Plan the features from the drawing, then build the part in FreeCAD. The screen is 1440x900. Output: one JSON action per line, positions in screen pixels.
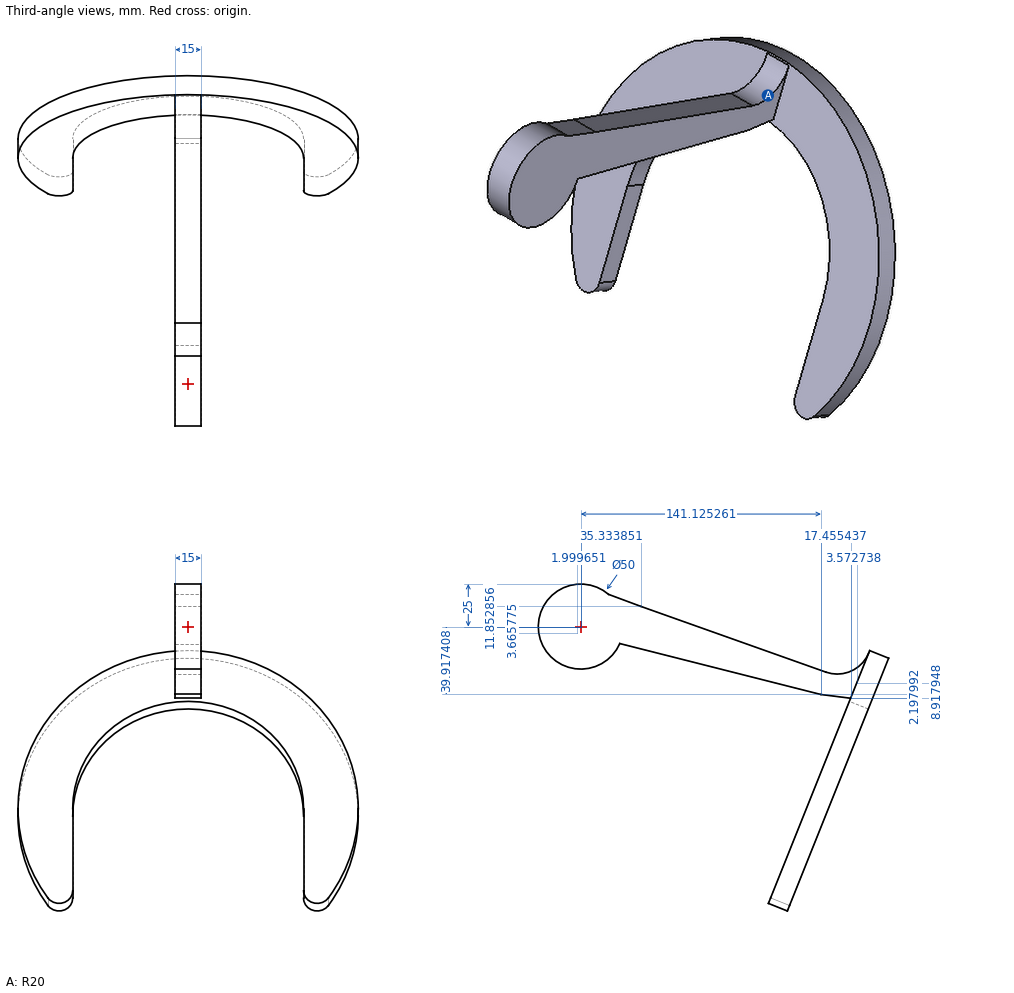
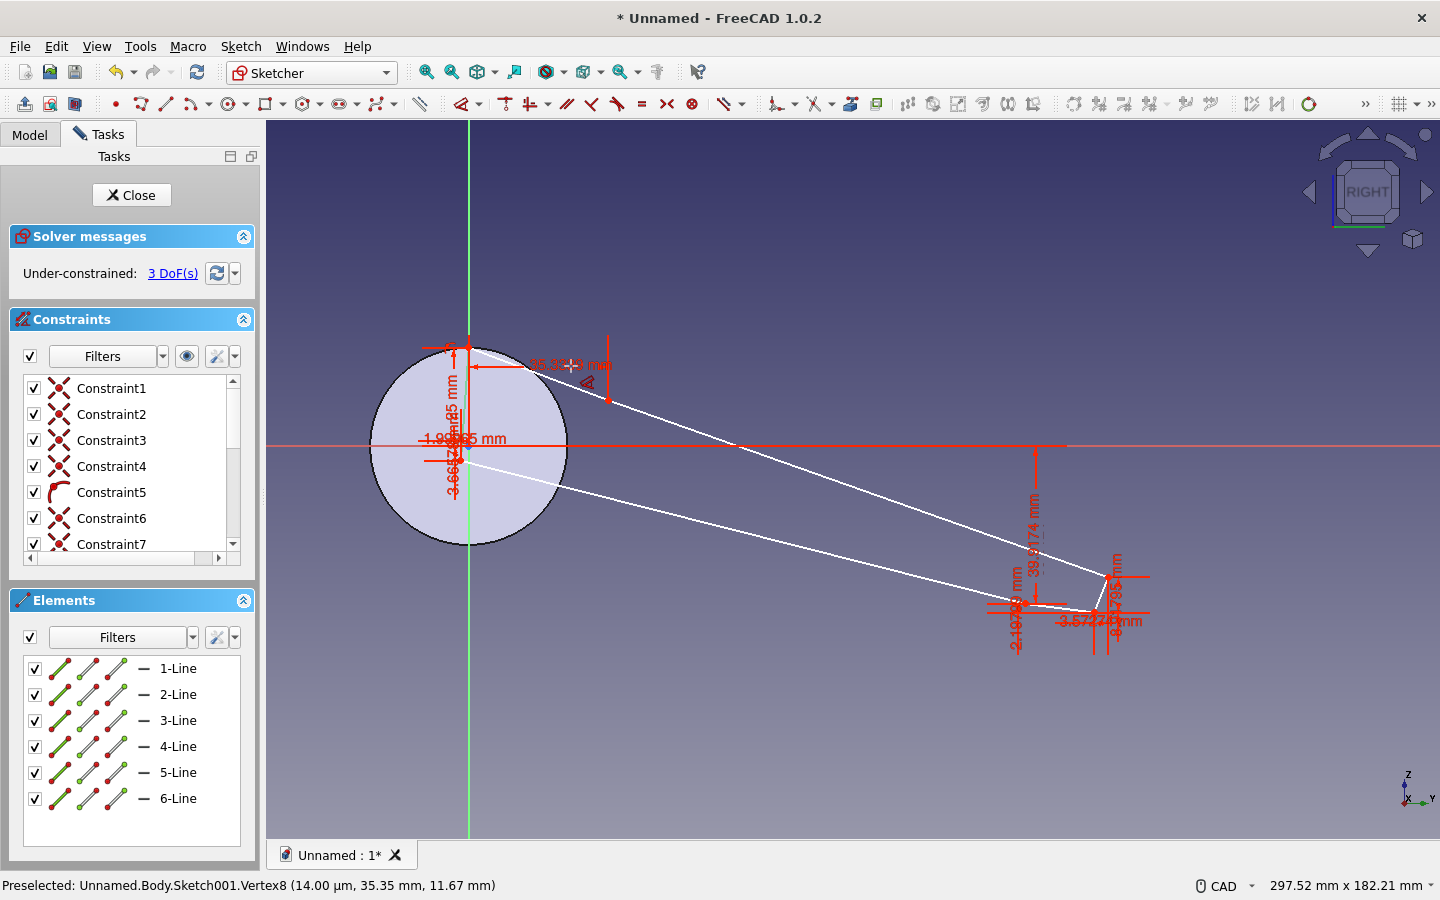
{"action": "left_click", "coordinate": [608, 400]}
{"action": "left_click", "coordinate": [387, 423]}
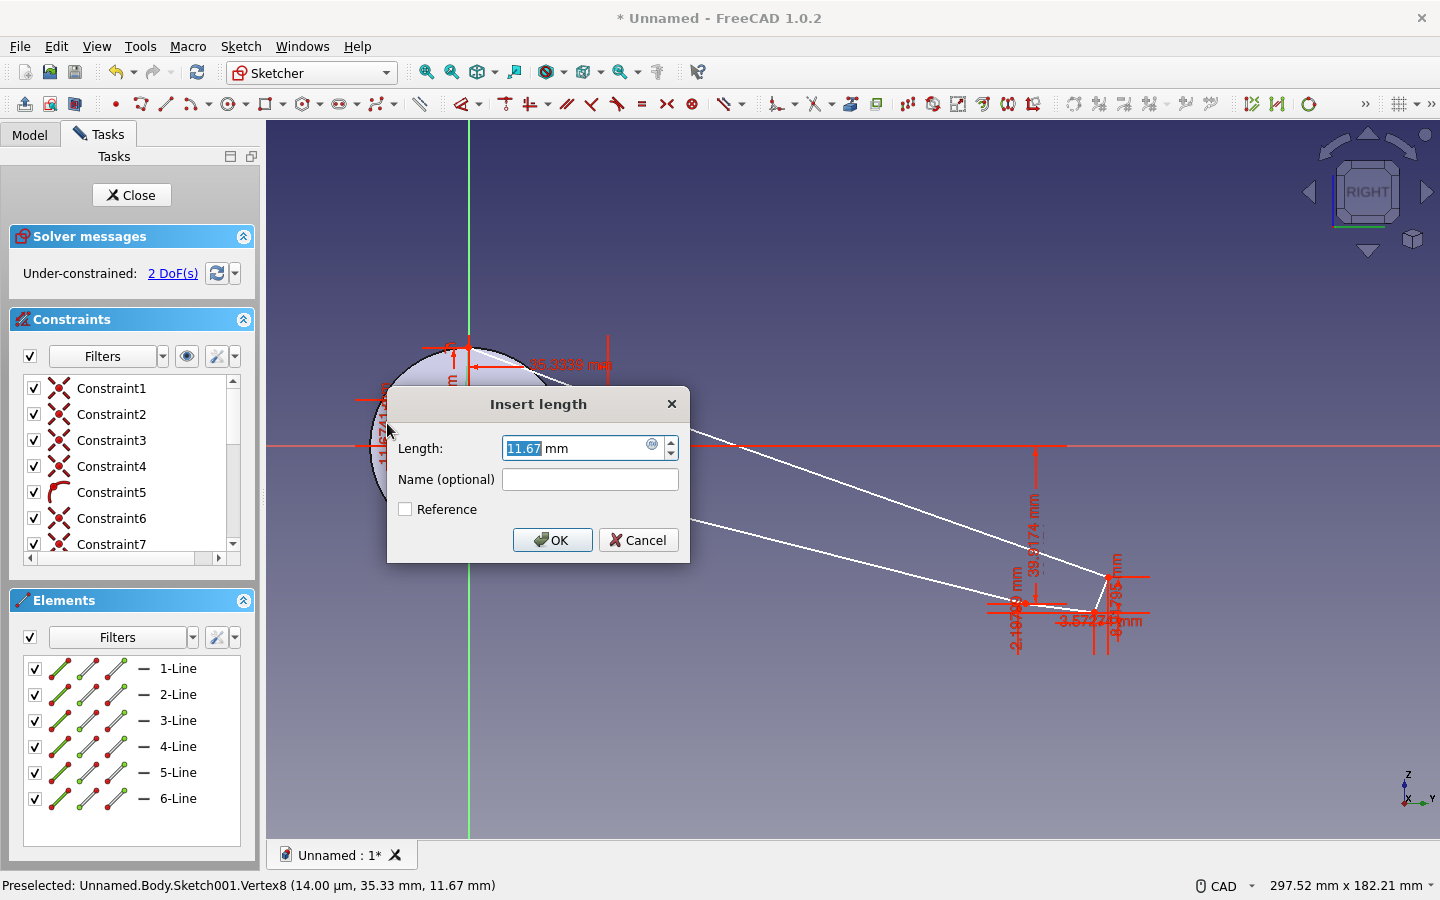
{"action": "type", "text": "11.852856"}
{"action": "key", "text": "Return"}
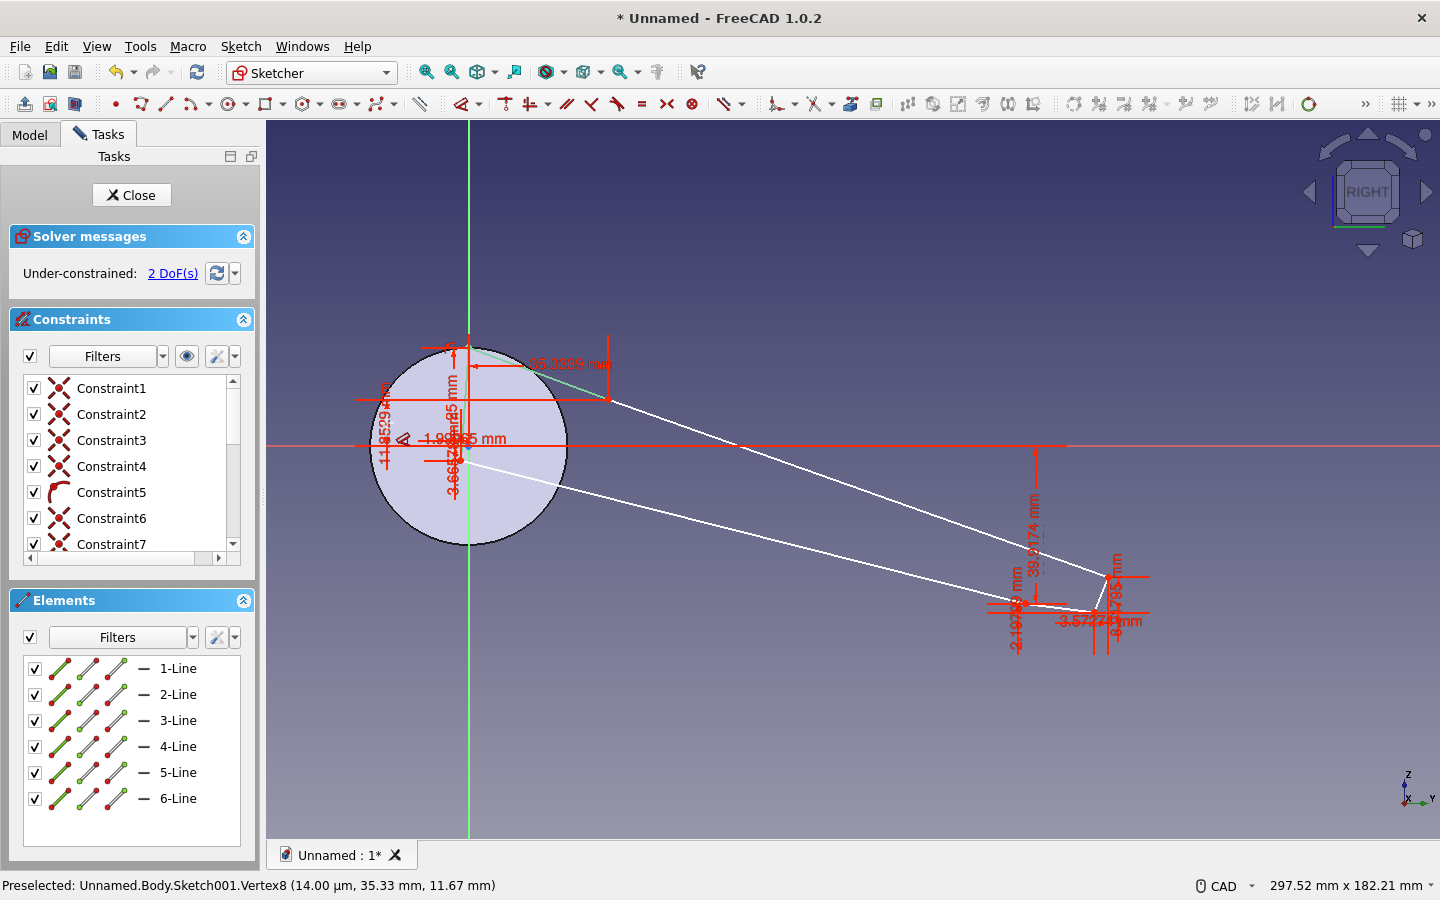
{"action": "left_click", "coordinate": [1046, 606]}
{"action": "left_click", "coordinate": [1060, 647]}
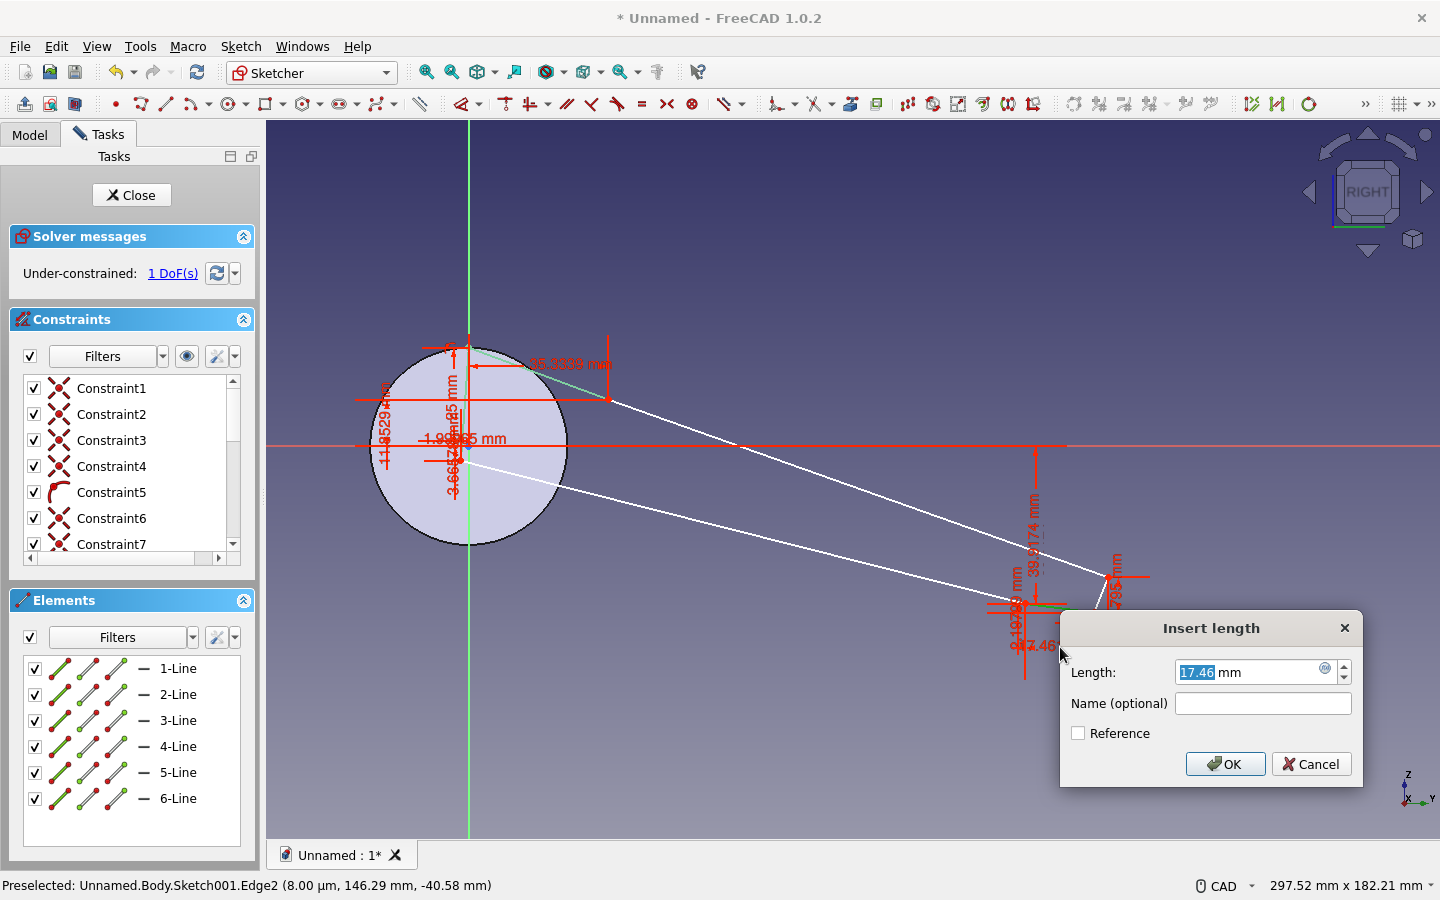
{"action": "type", "text": "17.455437"}
{"action": "key", "text": "Return"}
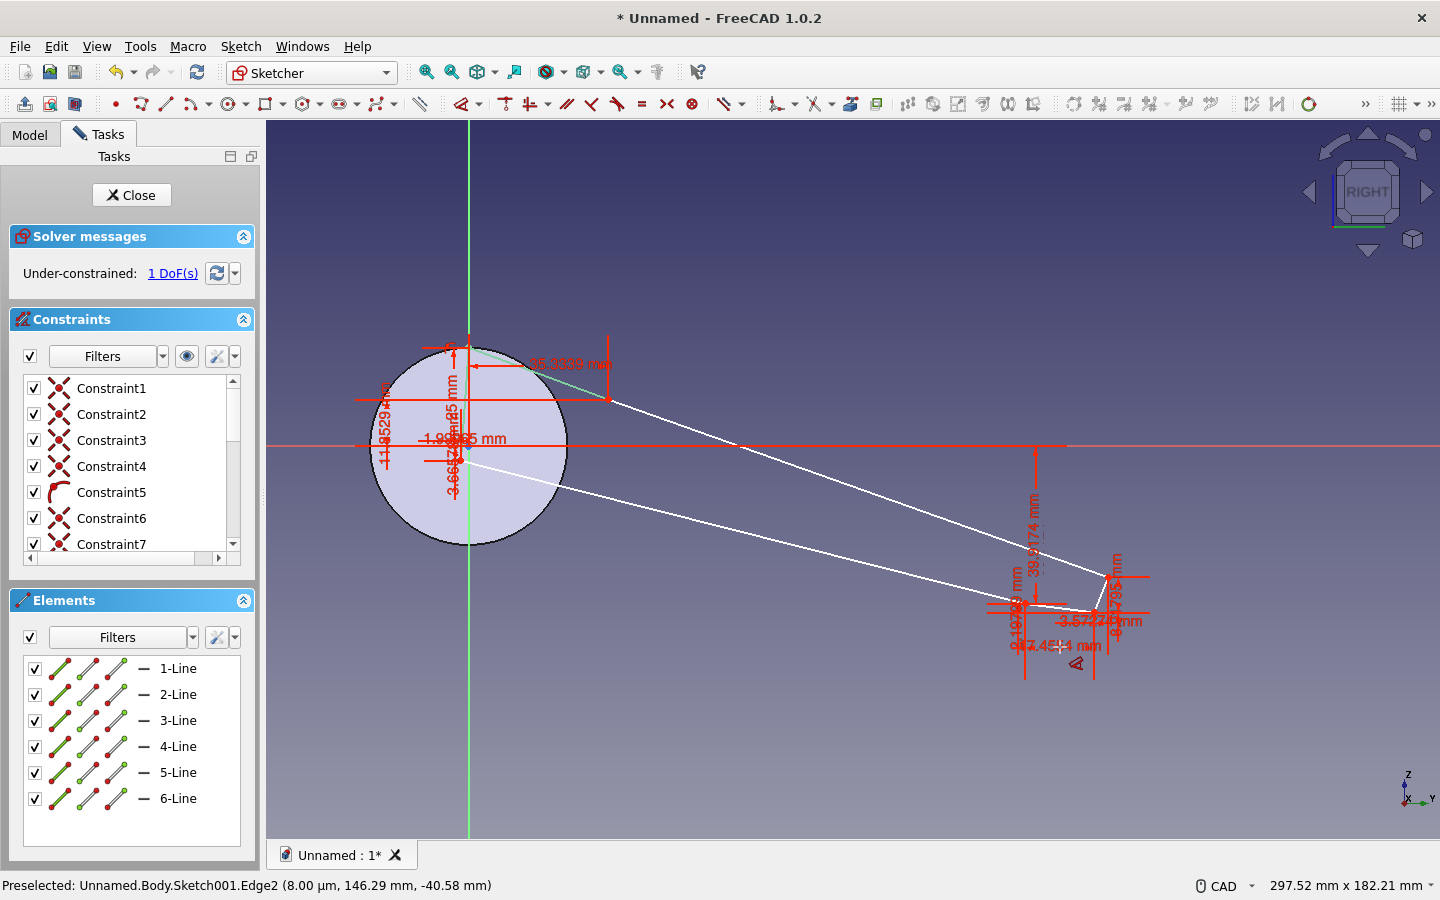
{"action": "left_click", "coordinate": [1025, 604]}
{"action": "left_click", "coordinate": [747, 638]}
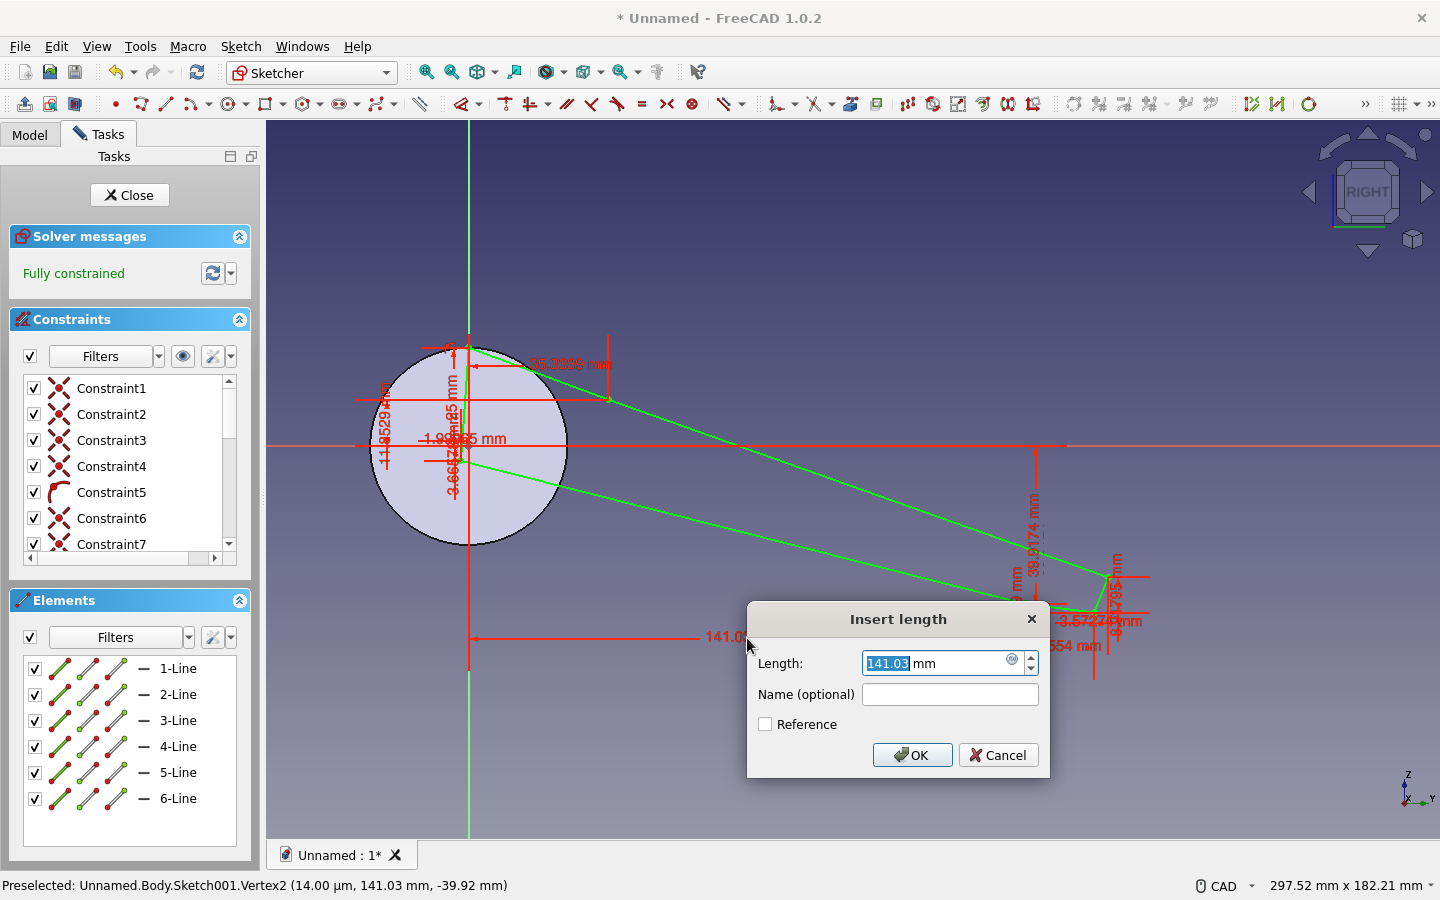
{"action": "type", "text": "141.125261"}
{"action": "key", "text": "Return"}
{"action": "key", "text": "Escape"}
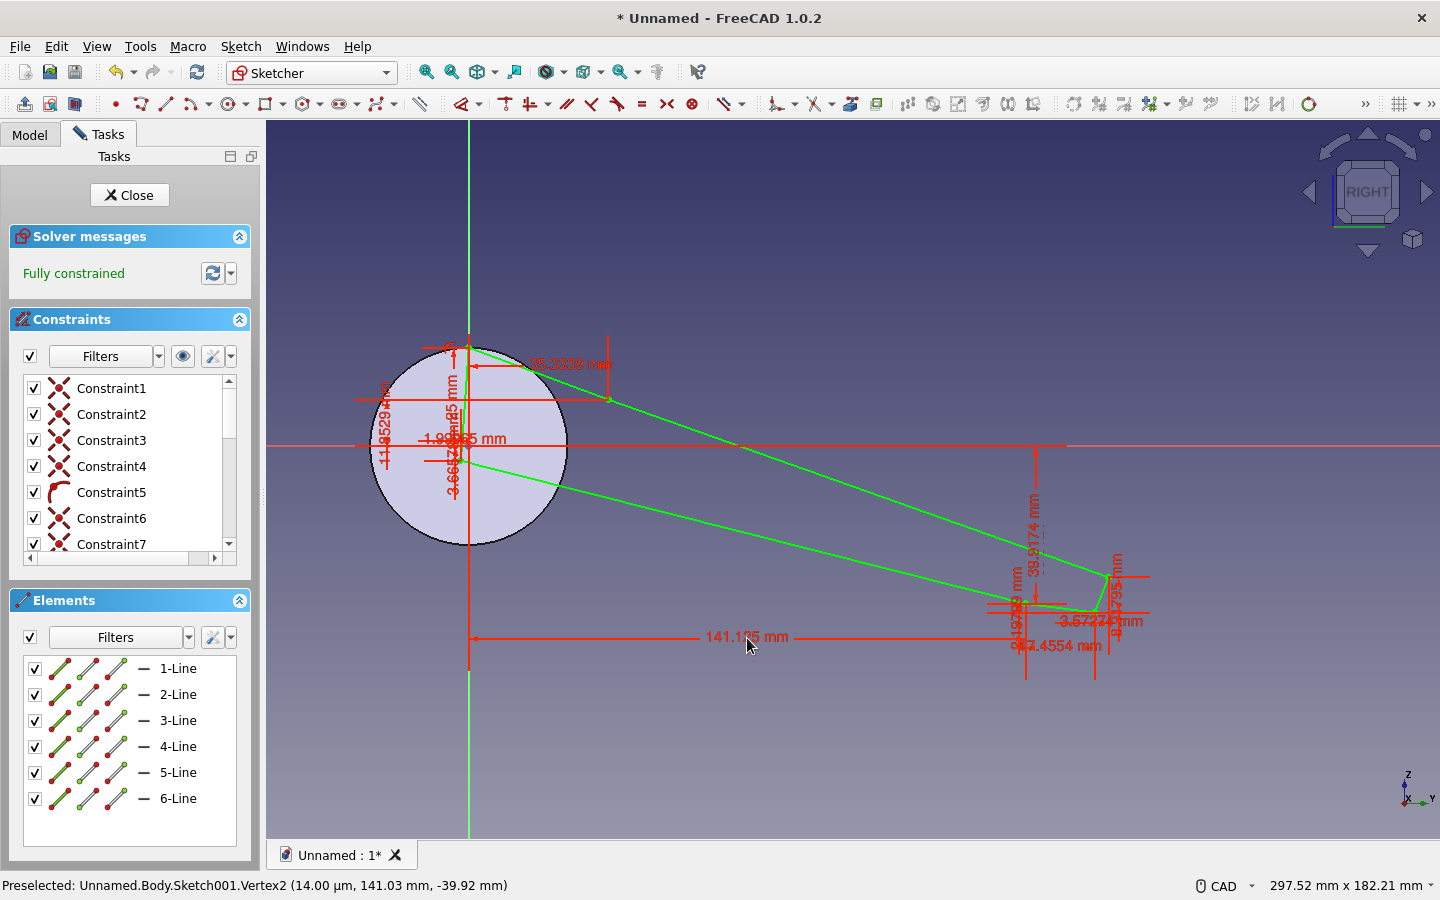
{"action": "left_click", "coordinate": [130, 195]}